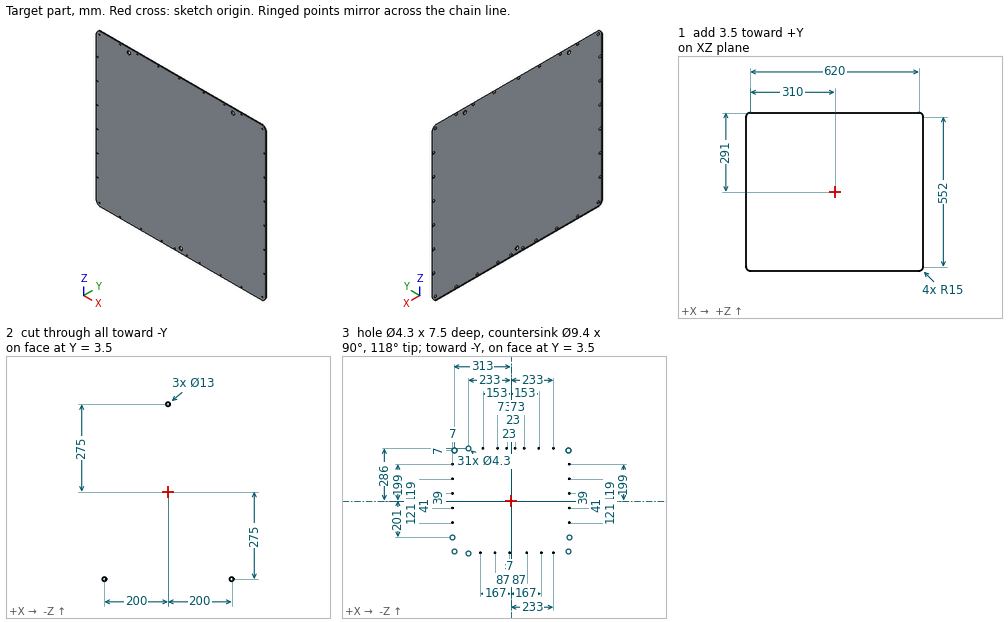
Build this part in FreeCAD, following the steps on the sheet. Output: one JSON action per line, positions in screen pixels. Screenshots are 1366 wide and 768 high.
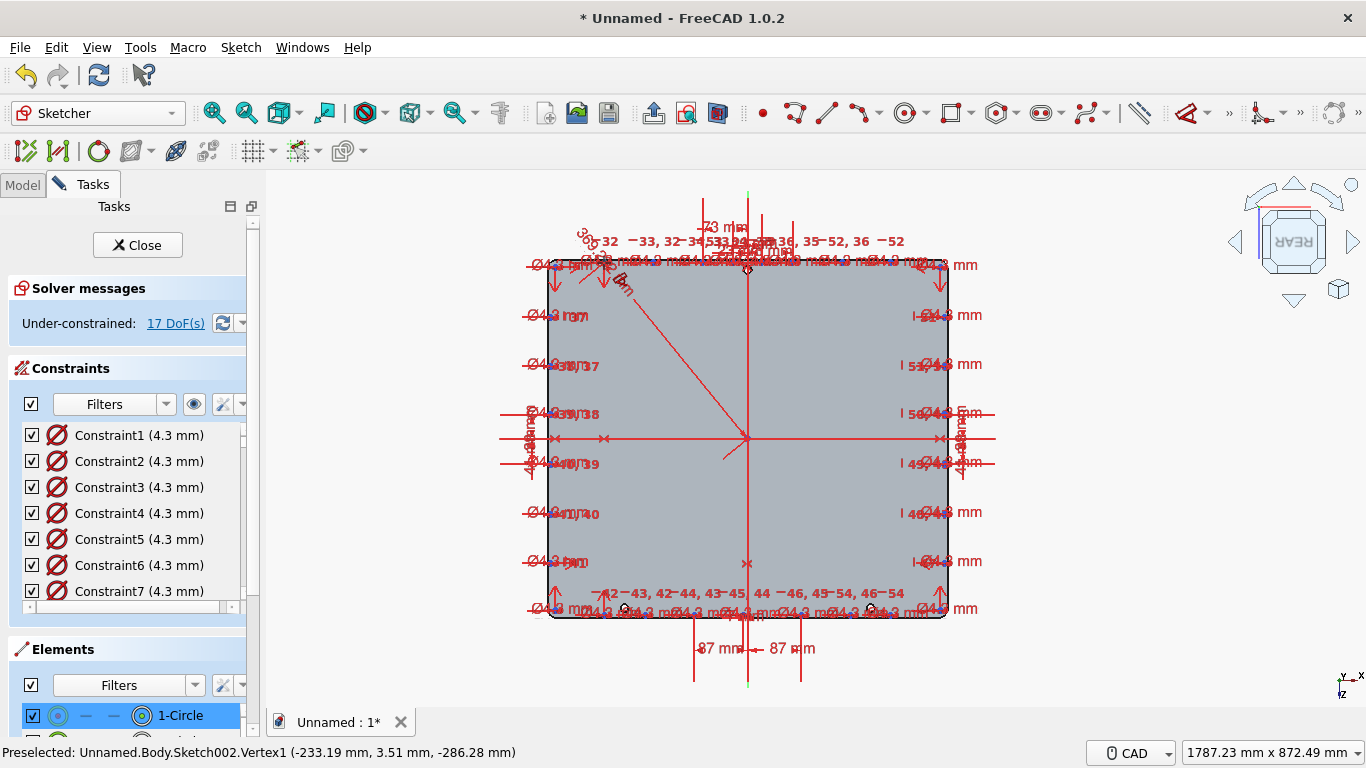
{"action": "scroll", "coordinate": [555, 267], "scroll_direction": "up", "scroll_amount": 12}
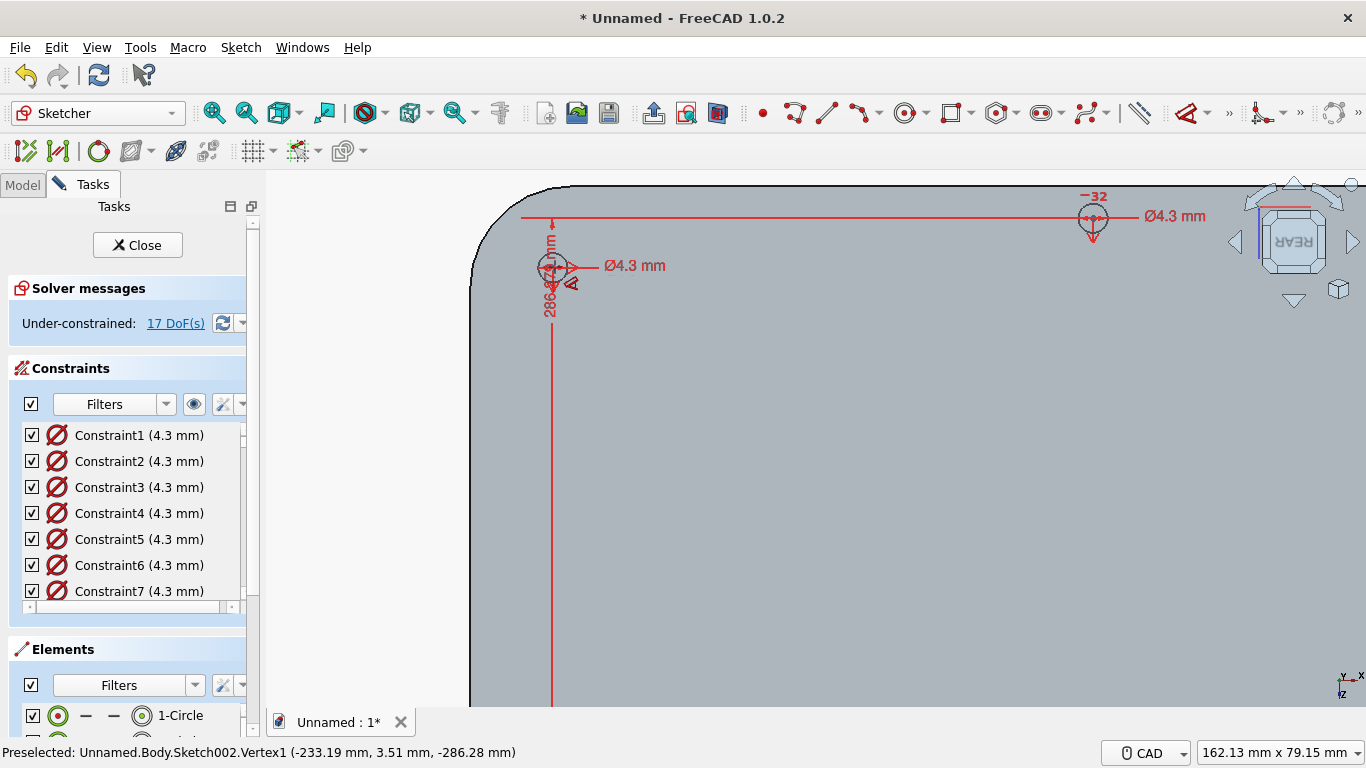
{"action": "left_click", "coordinate": [553, 268]}
{"action": "left_click", "coordinate": [519, 243]}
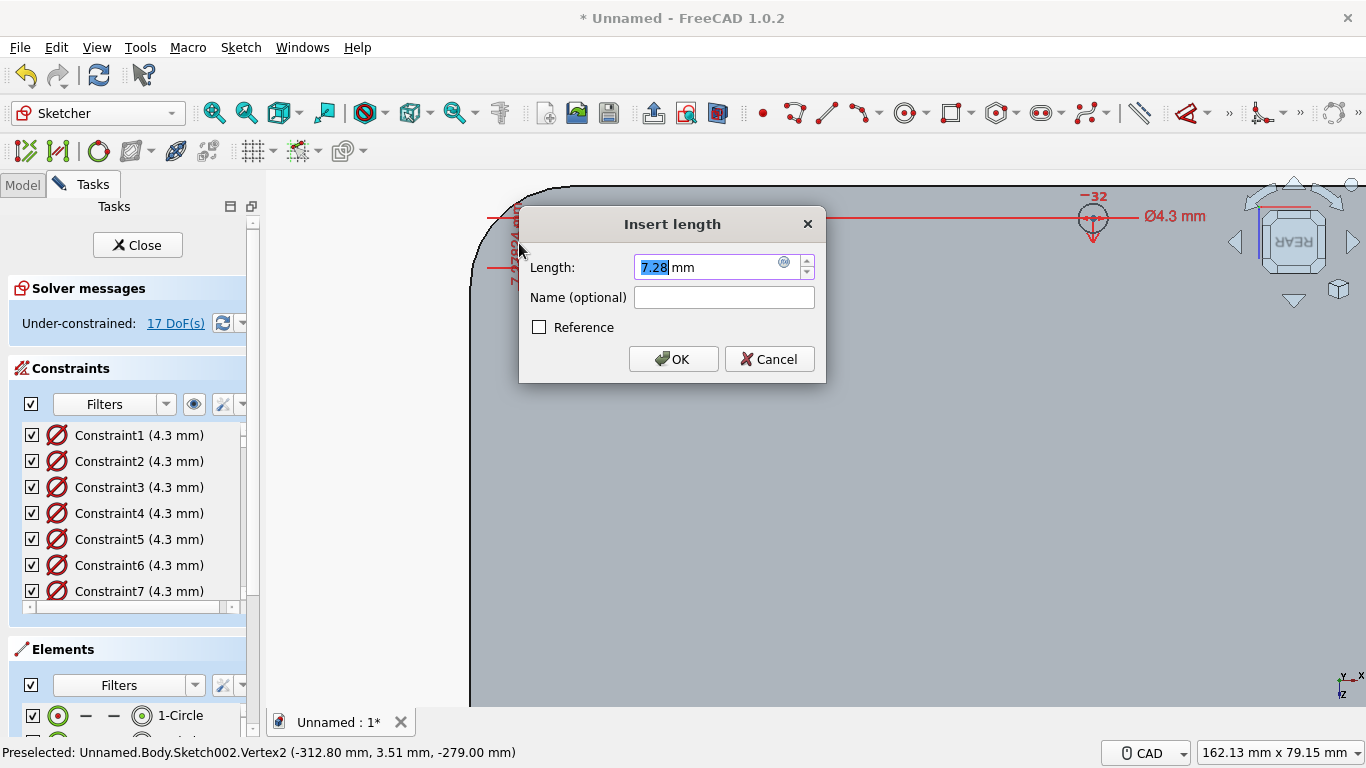
{"action": "type", "text": "7"}
{"action": "key", "text": "Return"}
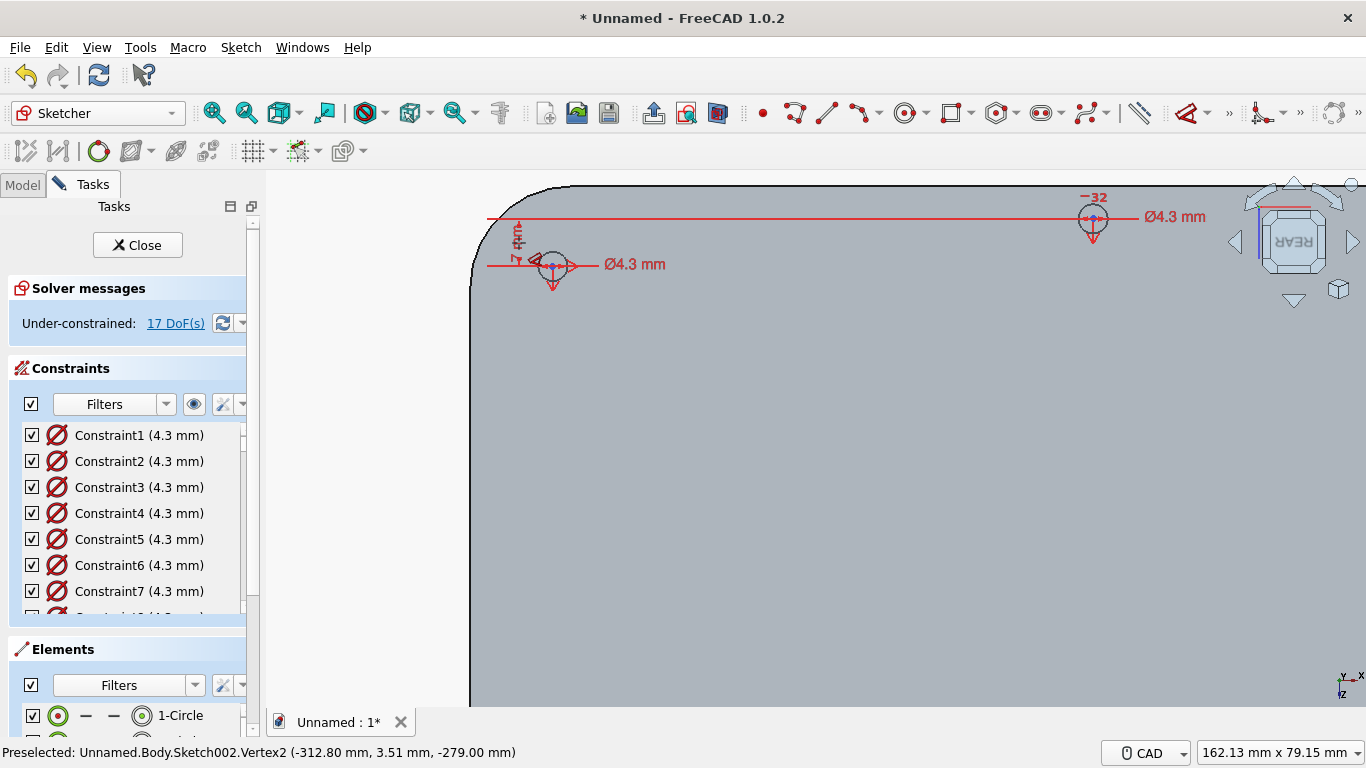
{"action": "left_click", "coordinate": [553, 266]}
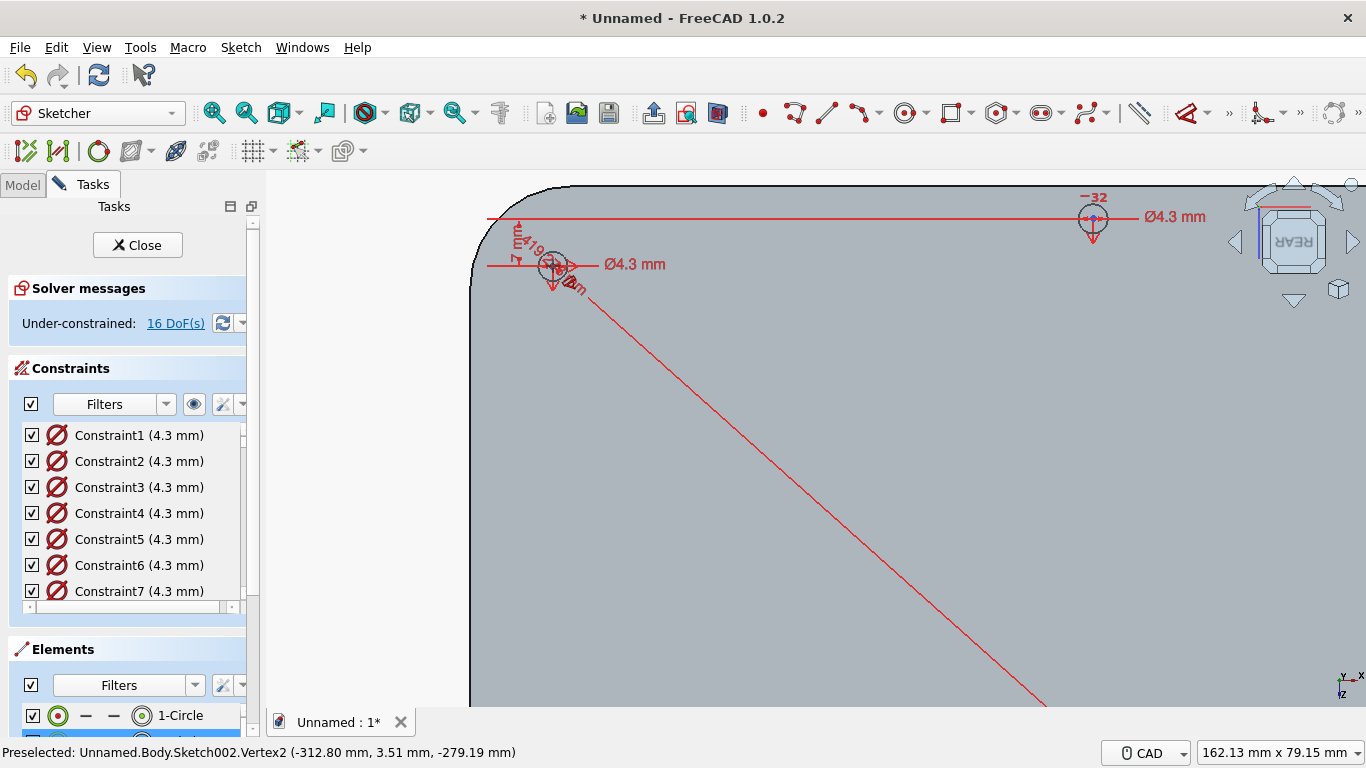
{"action": "scroll", "coordinate": [555, 267], "scroll_direction": "down", "scroll_amount": 12}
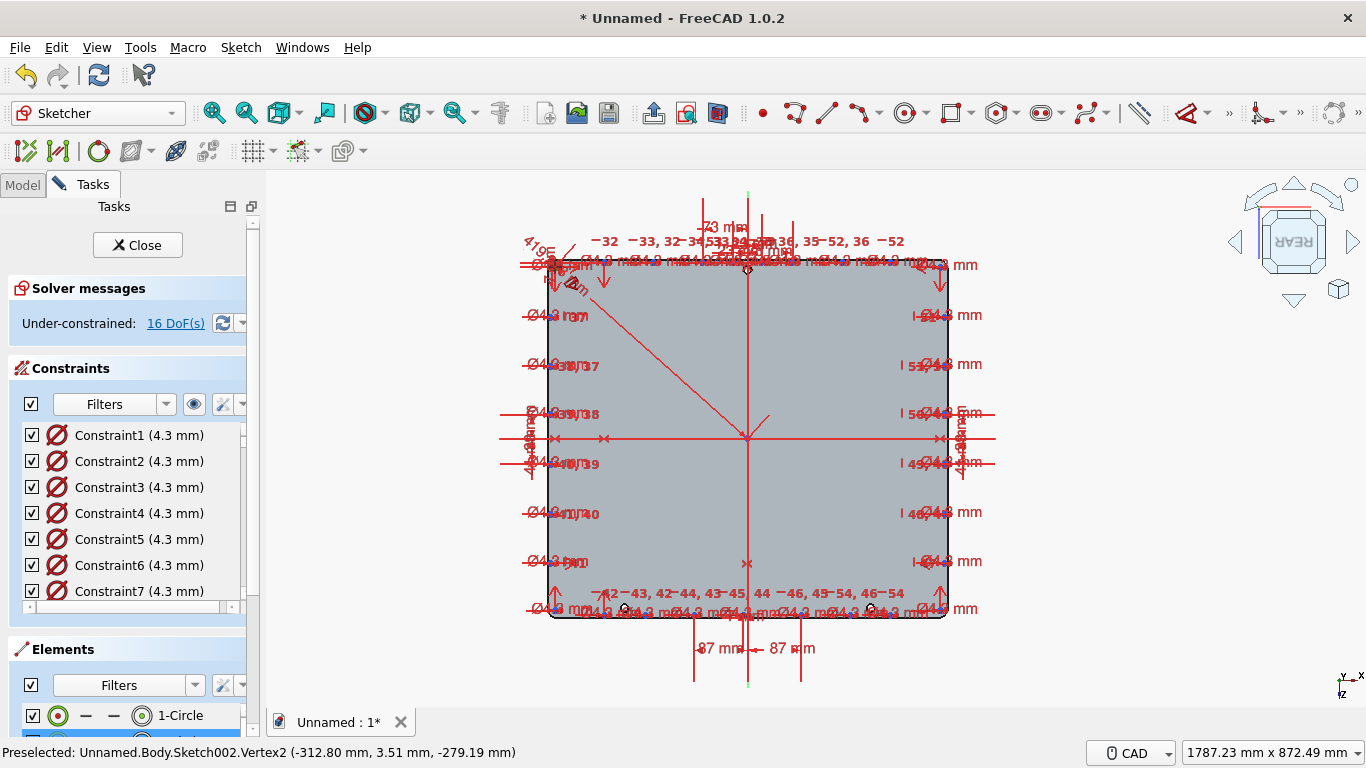
{"action": "scroll", "coordinate": [551, 317], "scroll_direction": "up", "scroll_amount": 12}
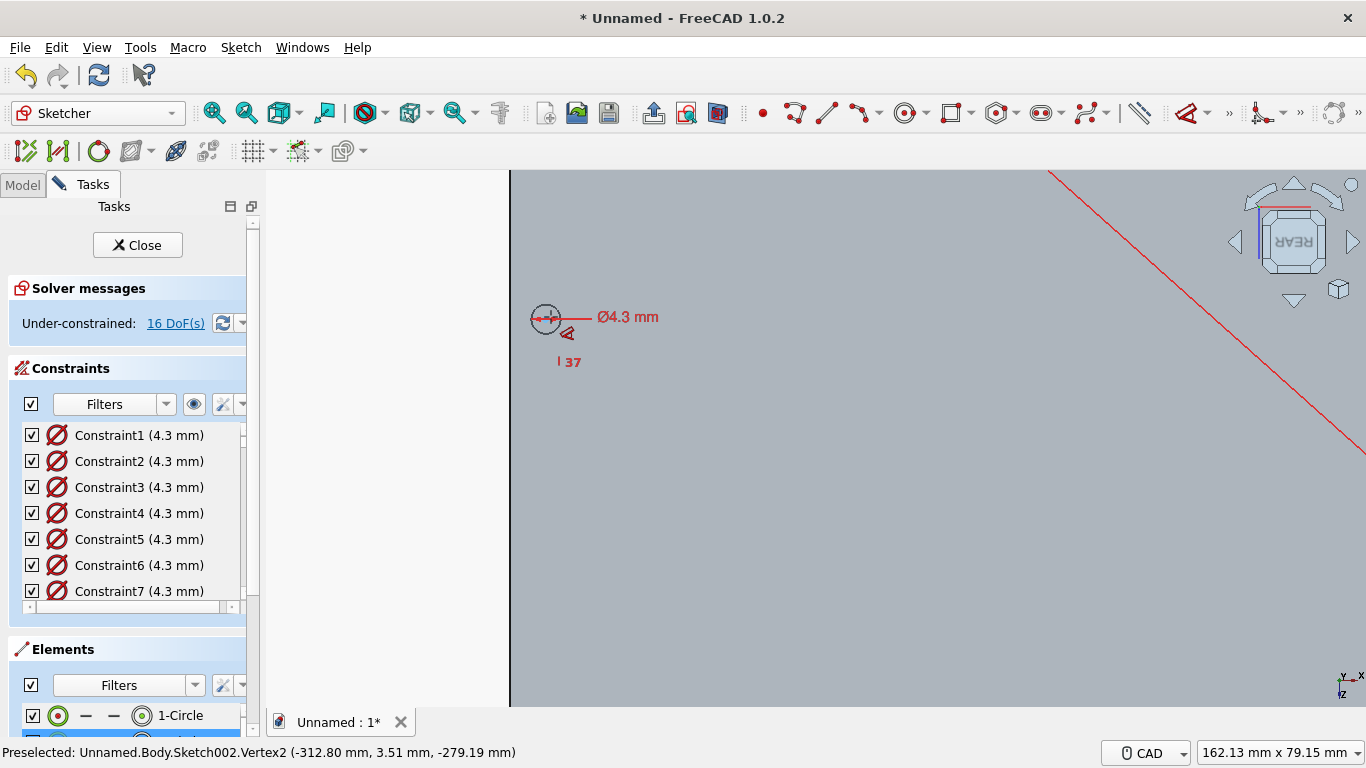
{"action": "left_click", "coordinate": [546, 319]}
{"action": "left_click", "coordinate": [570, 353]}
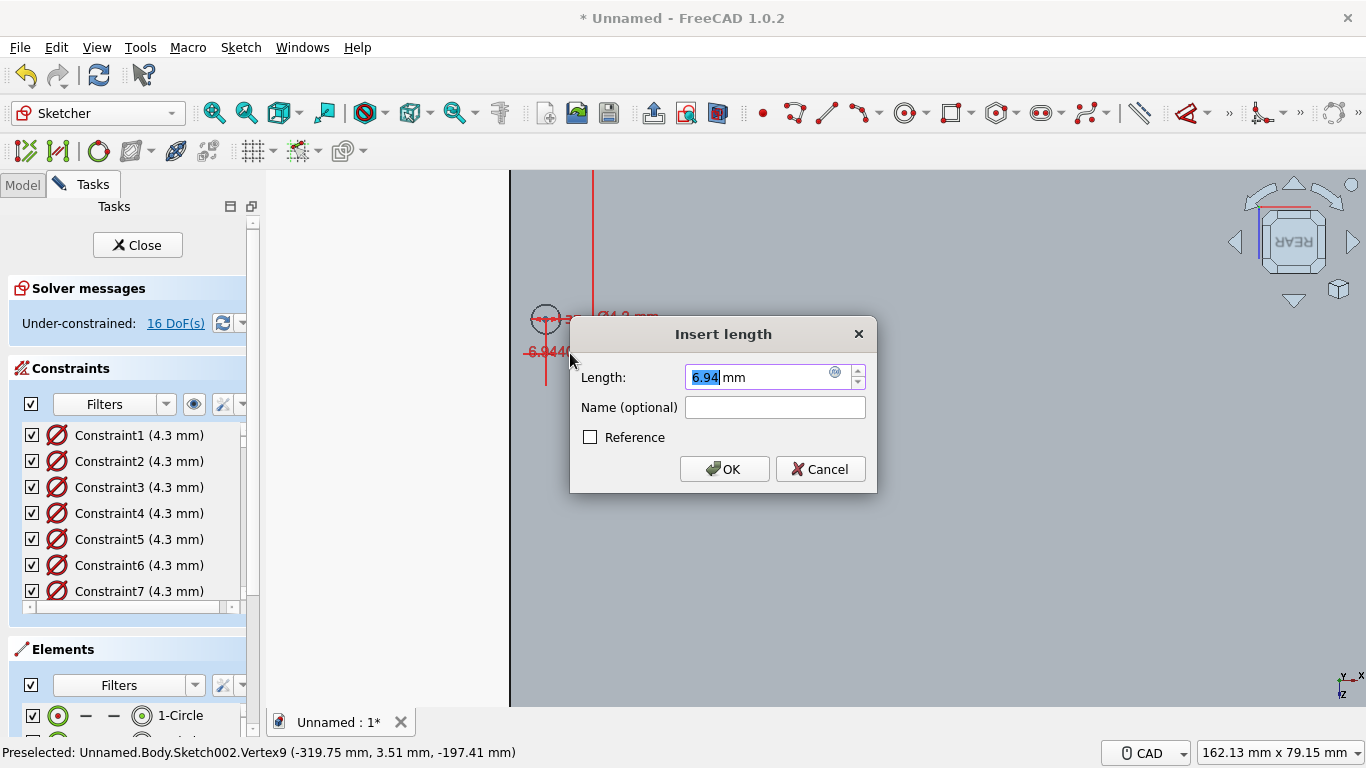
{"action": "type", "text": "7"}
{"action": "key", "text": "Return"}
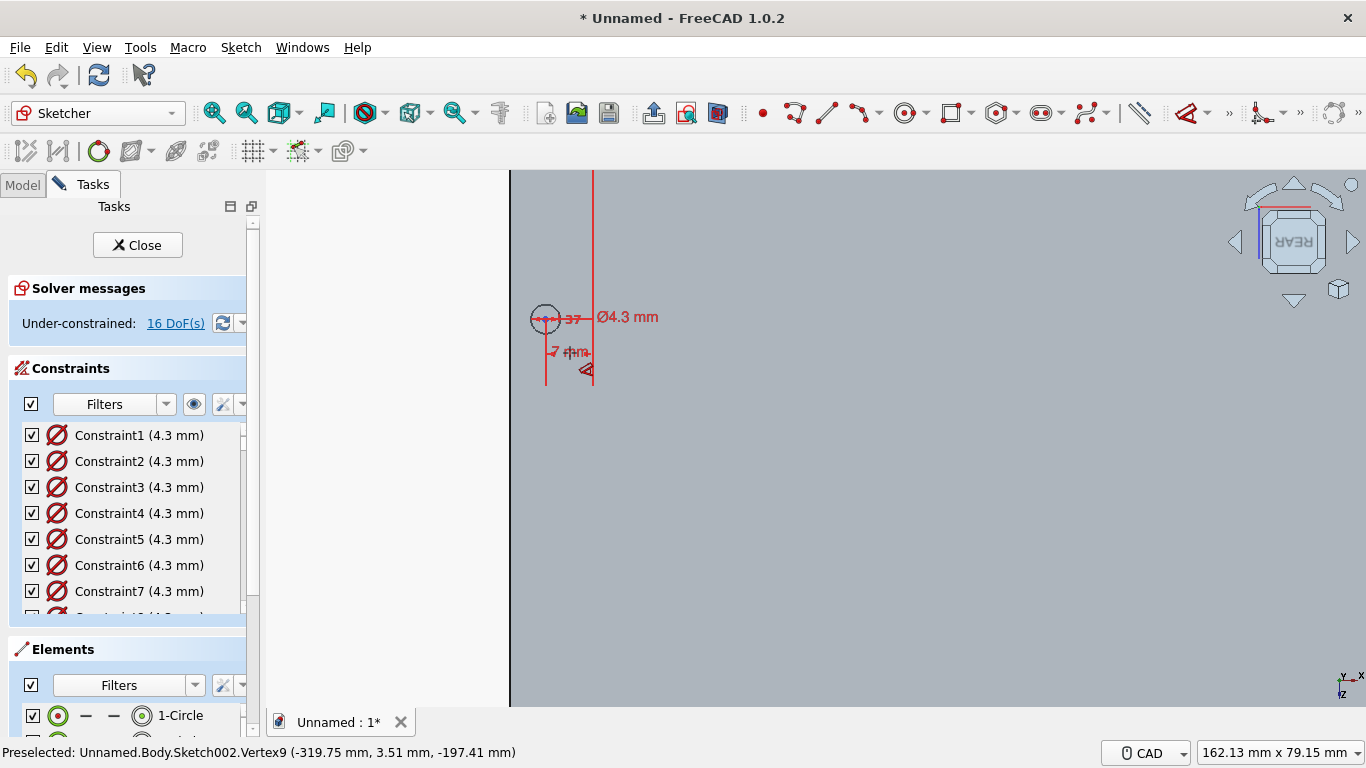
{"action": "scroll", "coordinate": [551, 317], "scroll_direction": "down", "scroll_amount": 12}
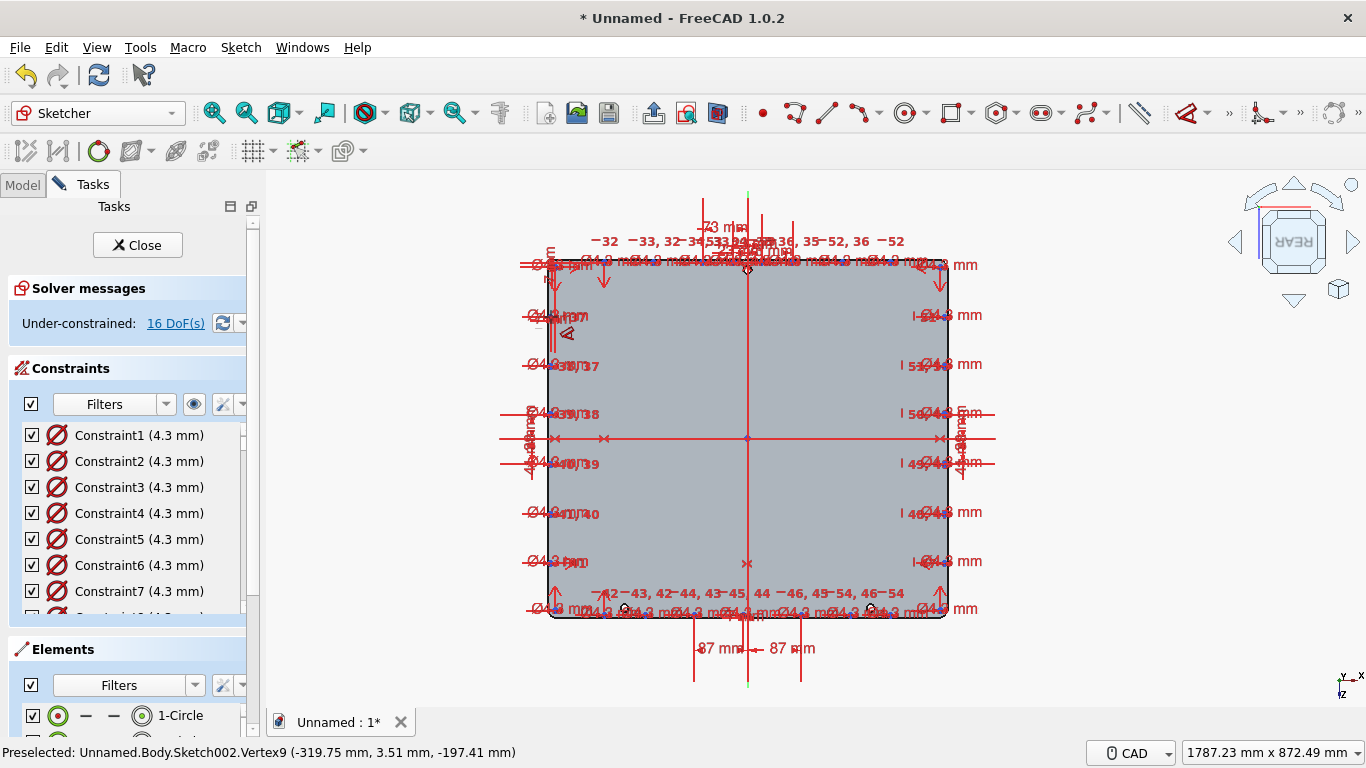
{"action": "left_click", "coordinate": [604, 263]}
{"action": "left_click", "coordinate": [643, 229]}